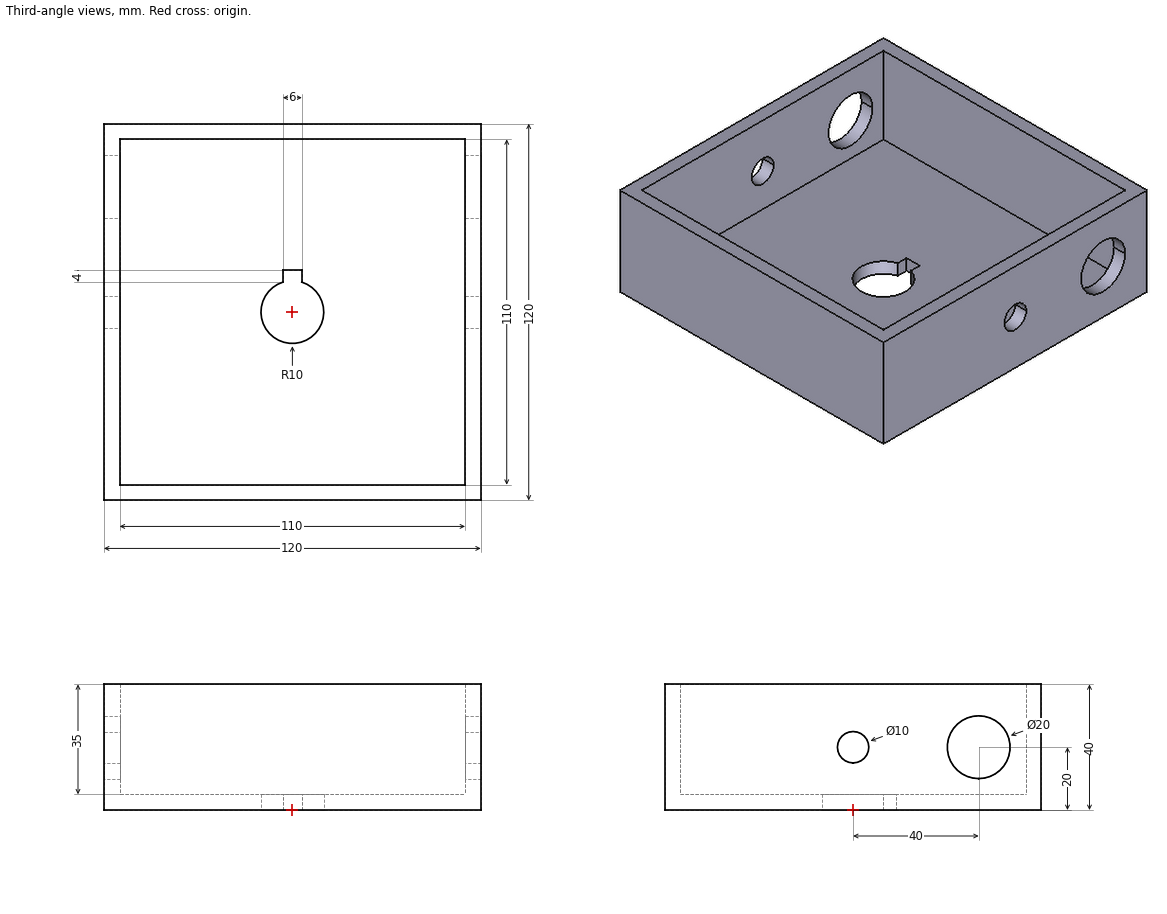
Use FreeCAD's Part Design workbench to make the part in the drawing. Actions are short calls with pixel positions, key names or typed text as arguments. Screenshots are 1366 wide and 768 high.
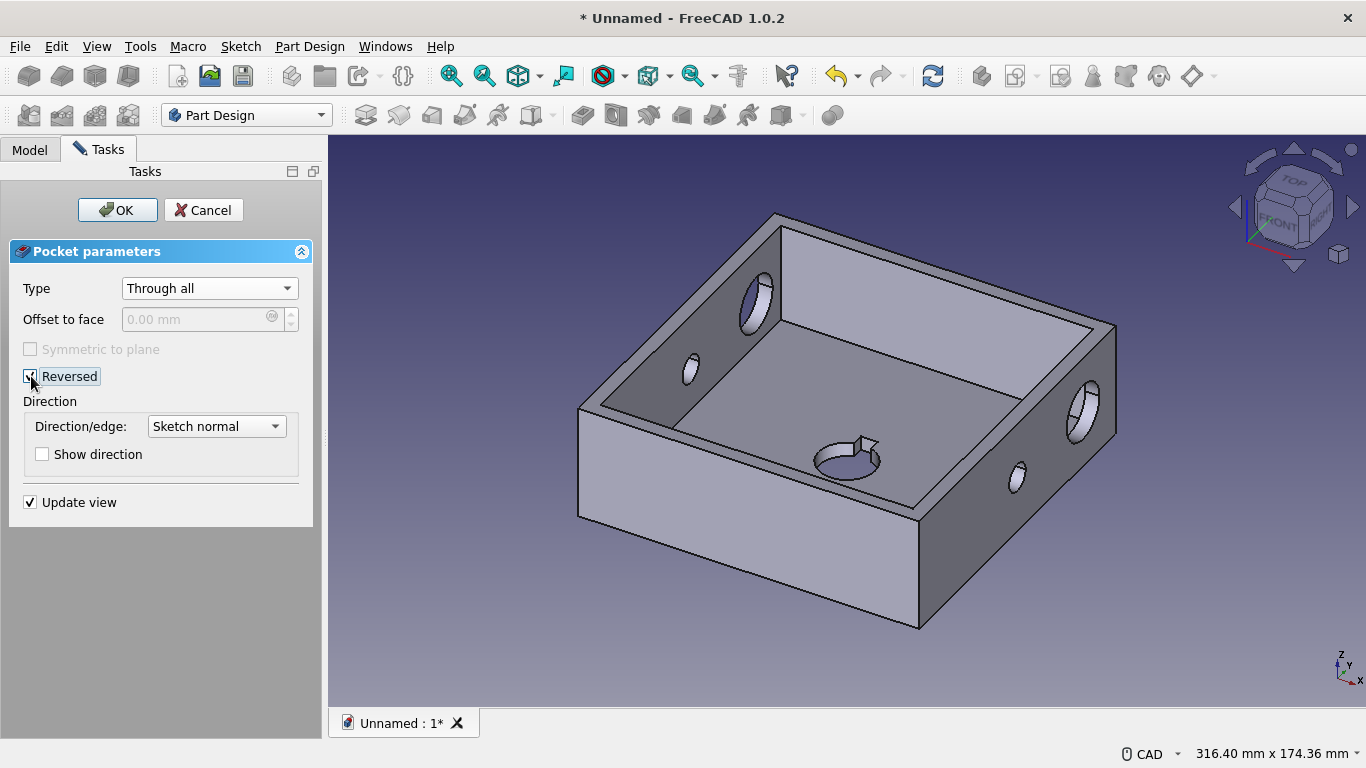
click(118, 210)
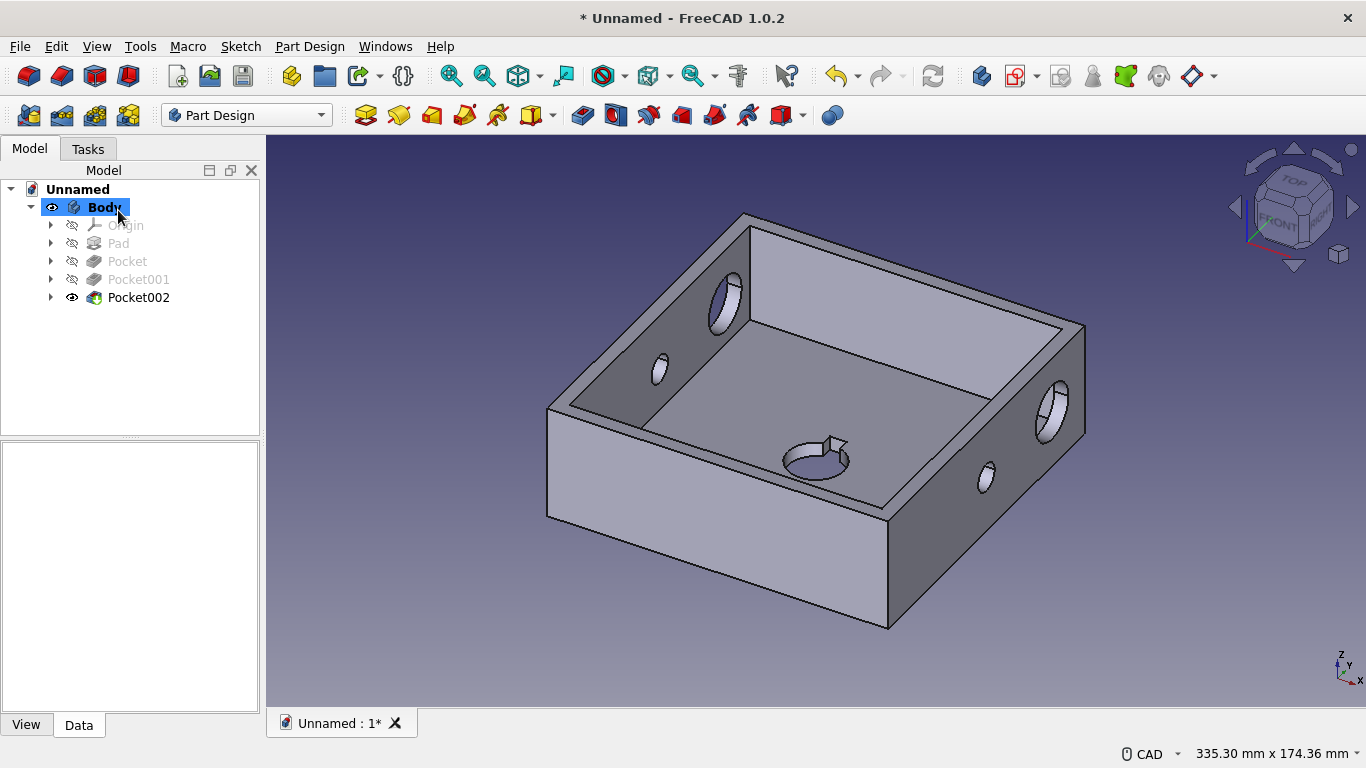
key(0)